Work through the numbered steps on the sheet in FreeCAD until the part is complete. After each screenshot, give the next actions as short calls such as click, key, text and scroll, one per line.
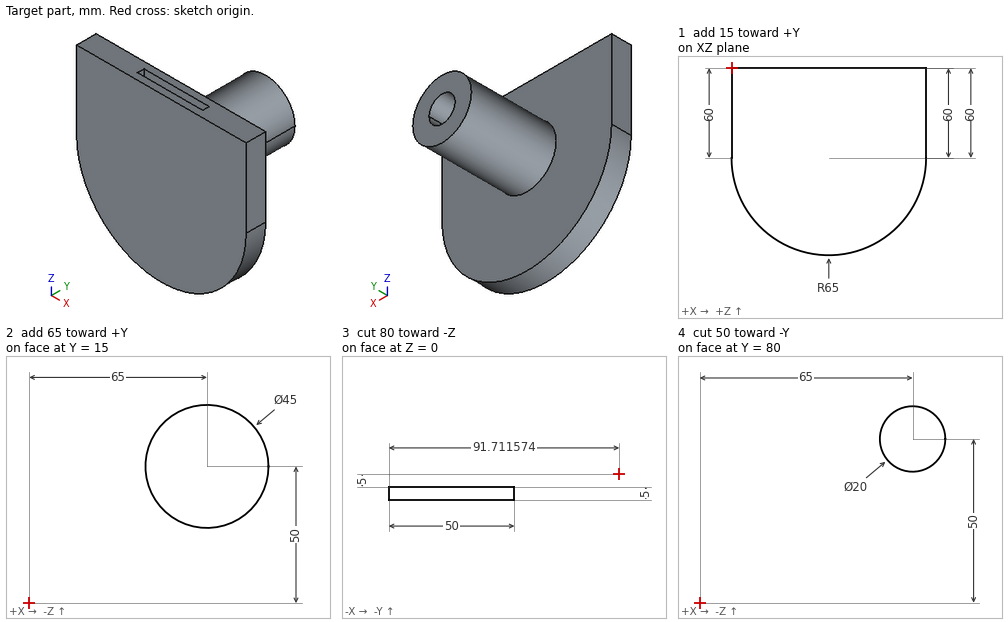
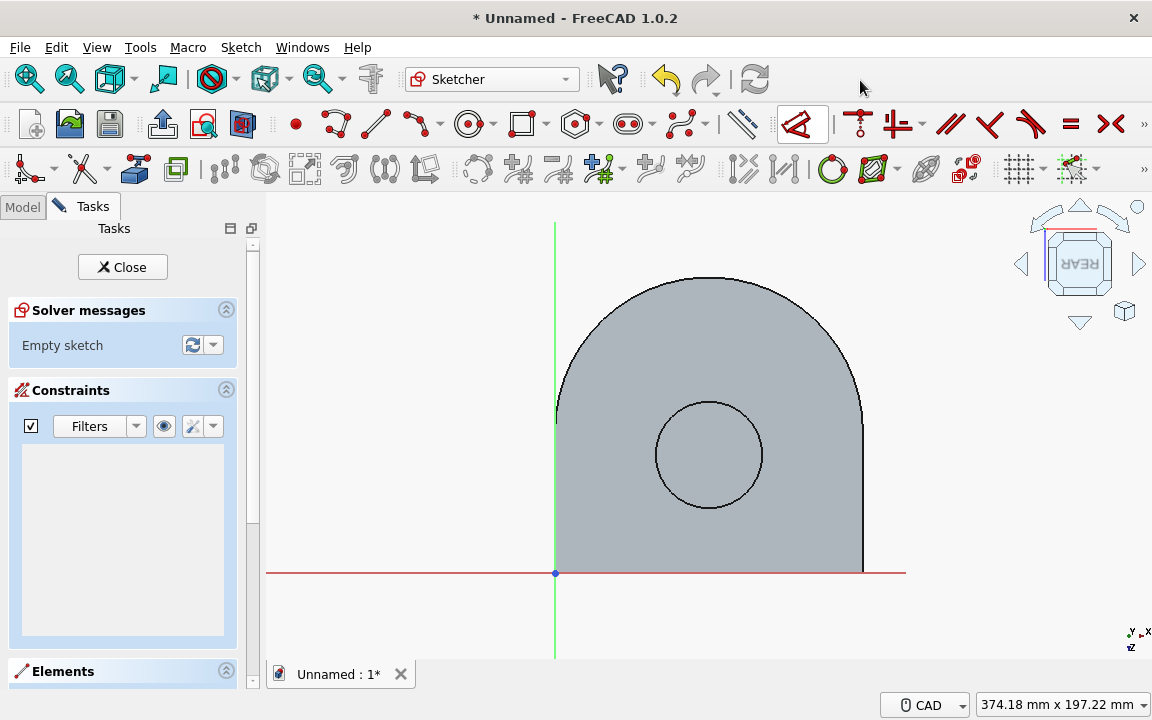
scroll(723, 461, up, 9)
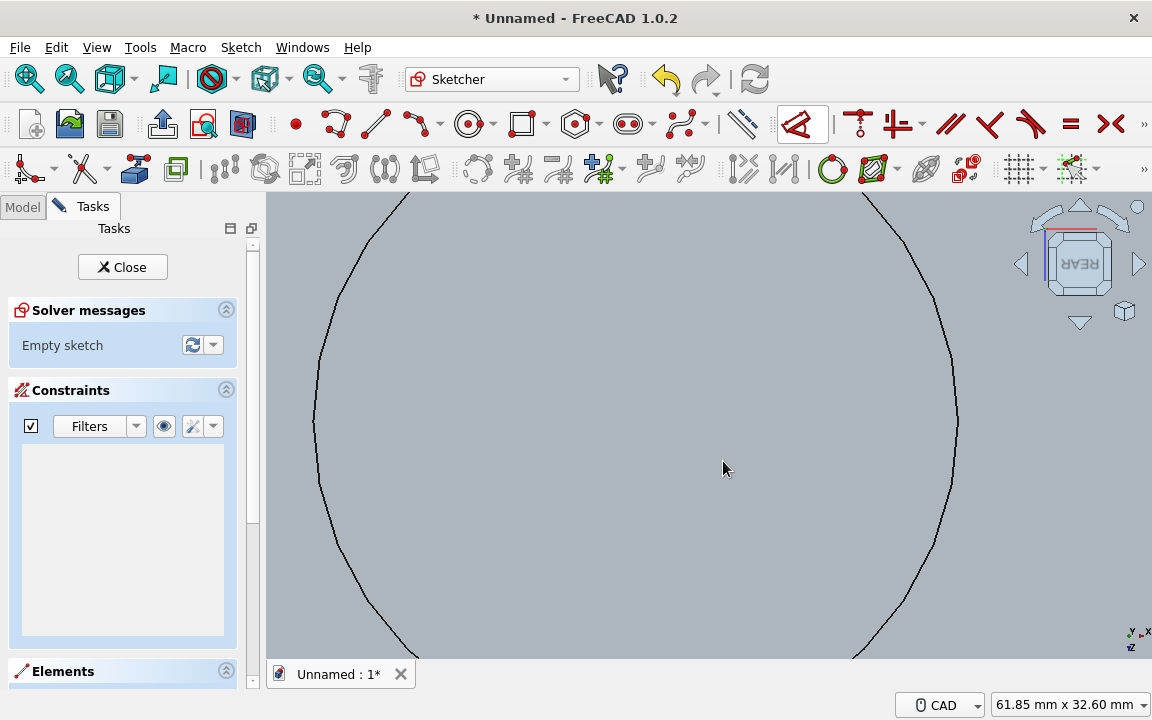
click(470, 124)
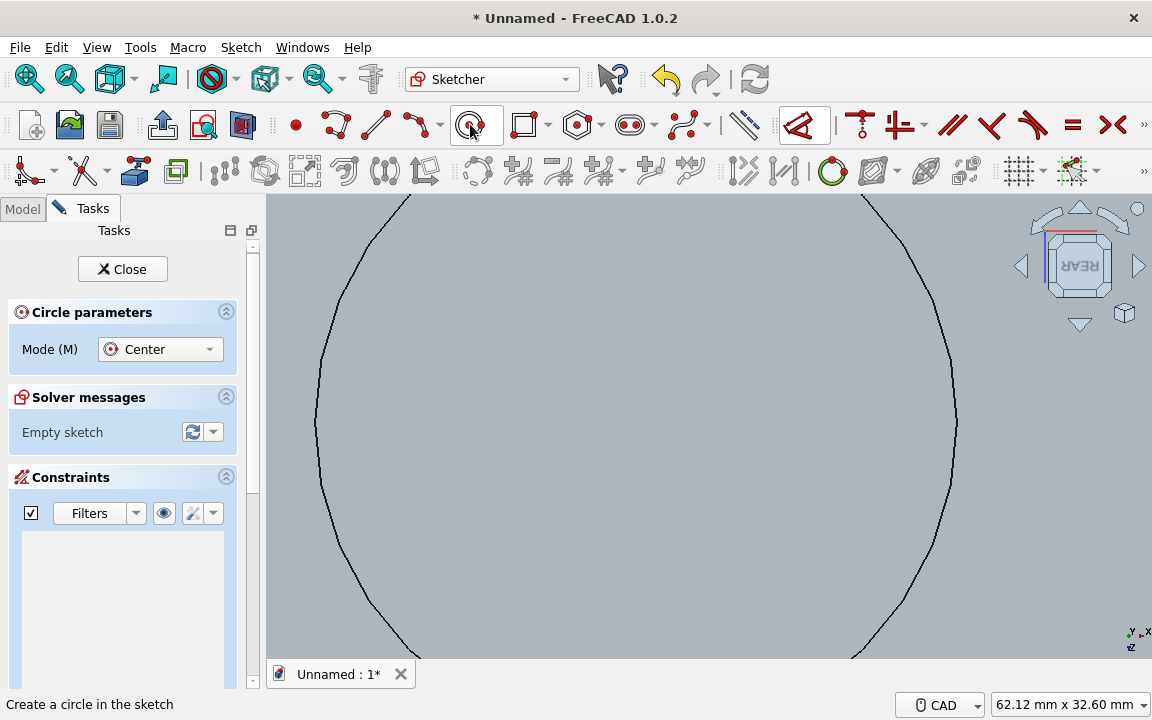
click(636, 423)
move(737, 322)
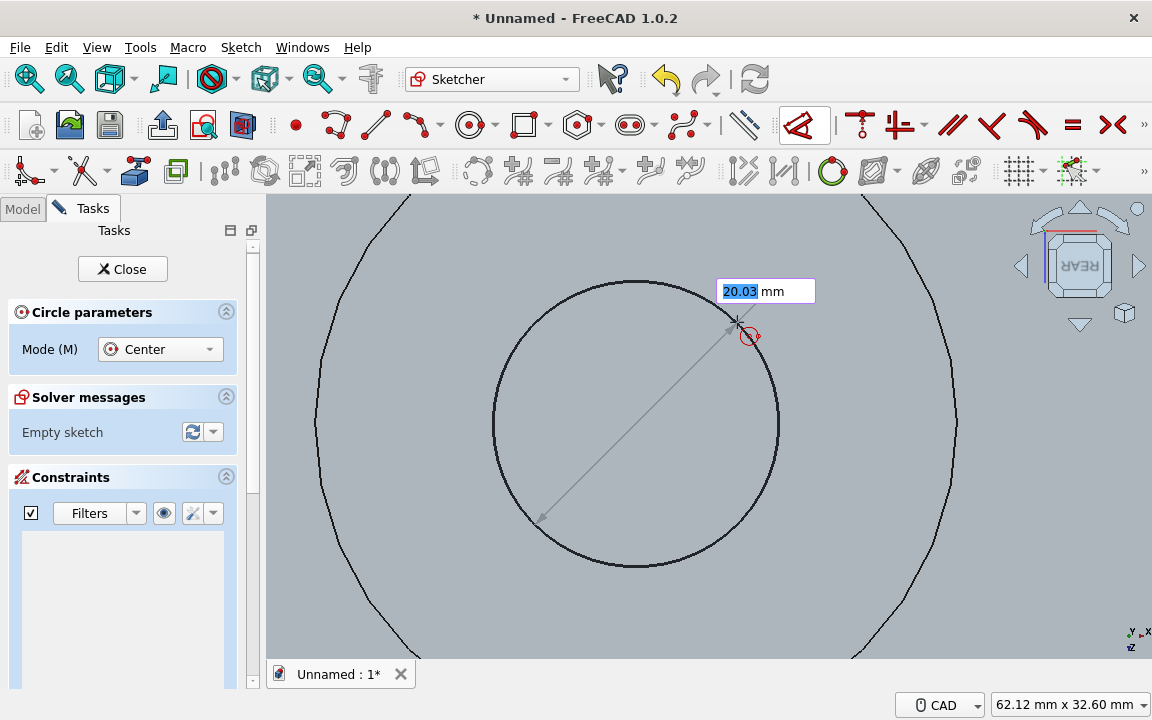
text(20)
key(Return)
key(Escape)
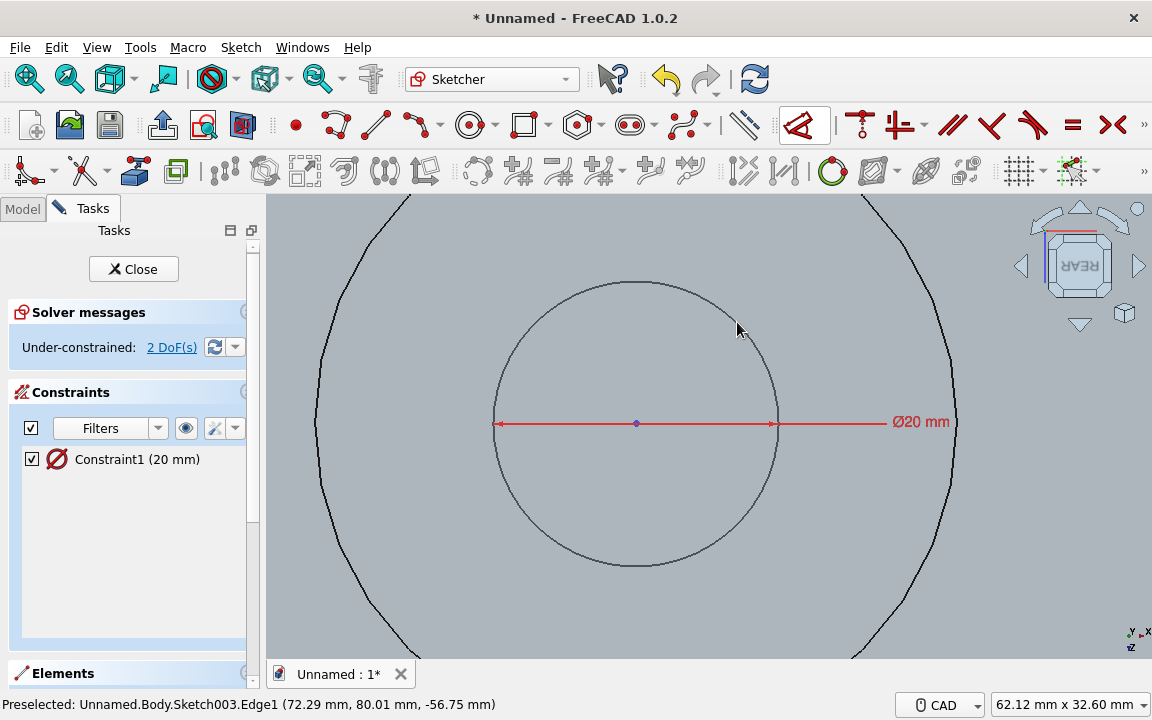
click(636, 424)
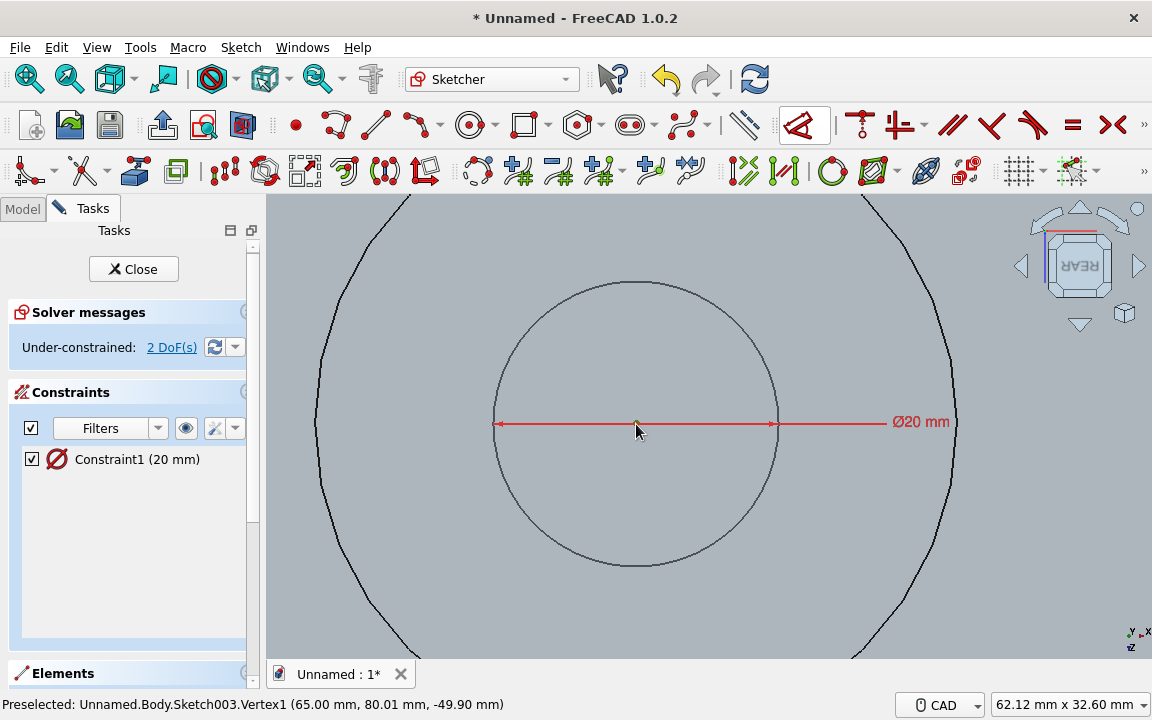
click(824, 126)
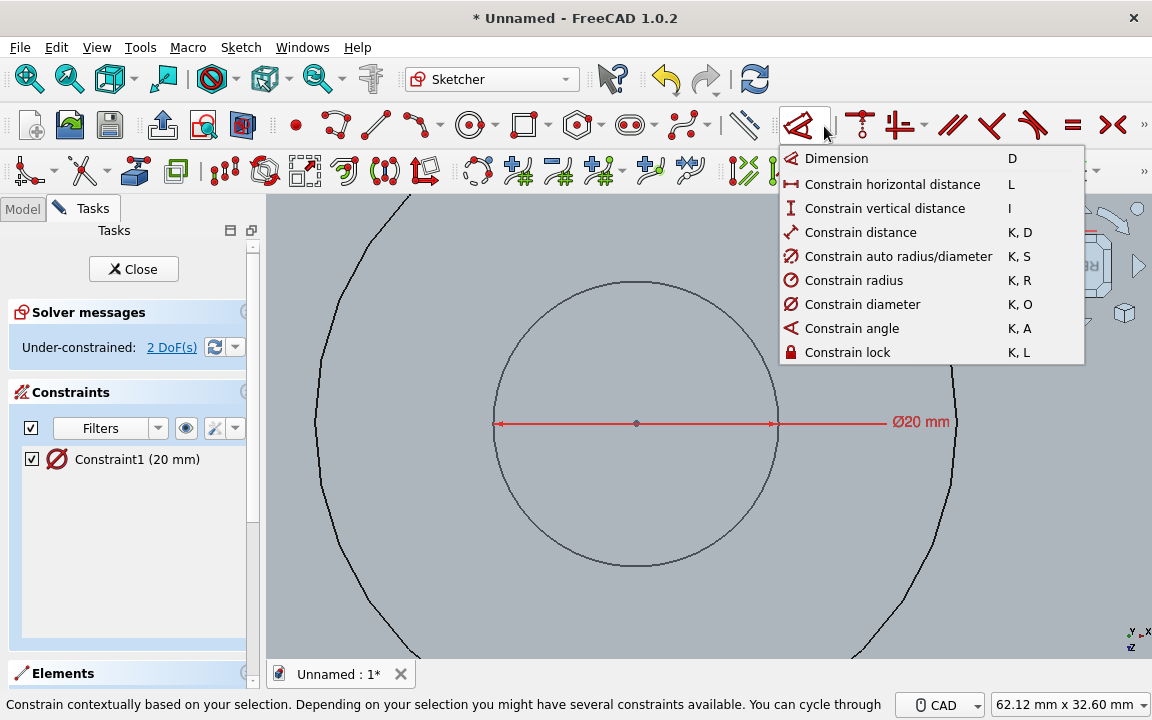
click(932, 184)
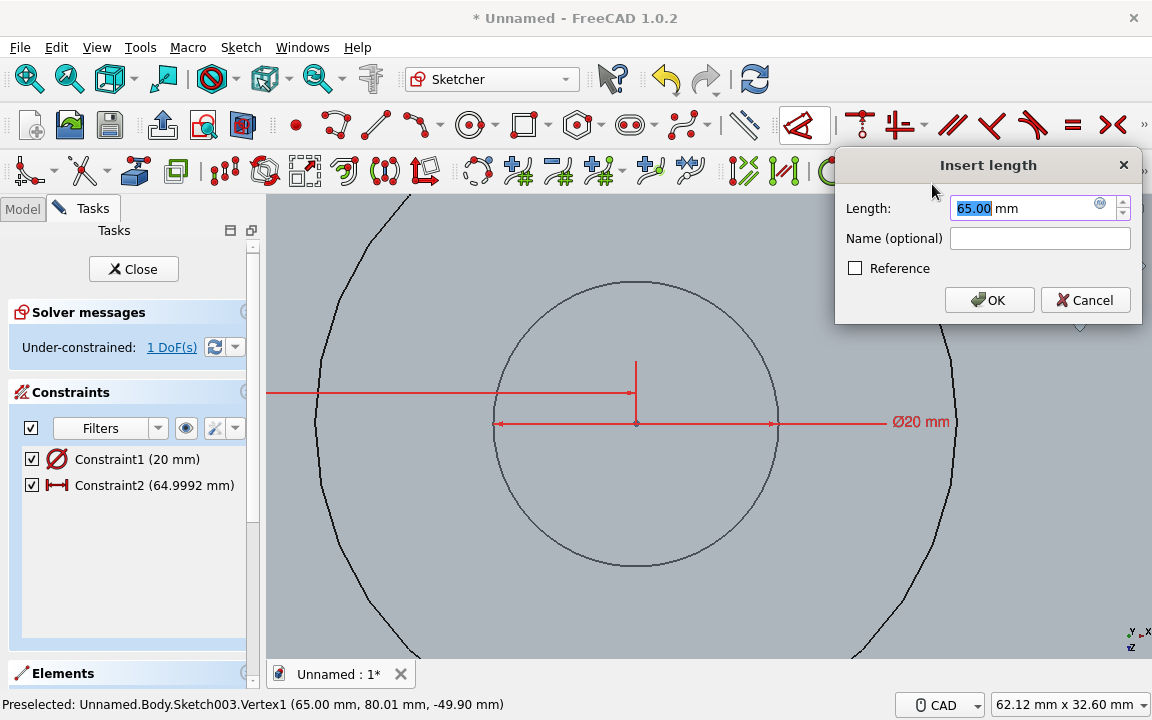
text(65)
key(Return)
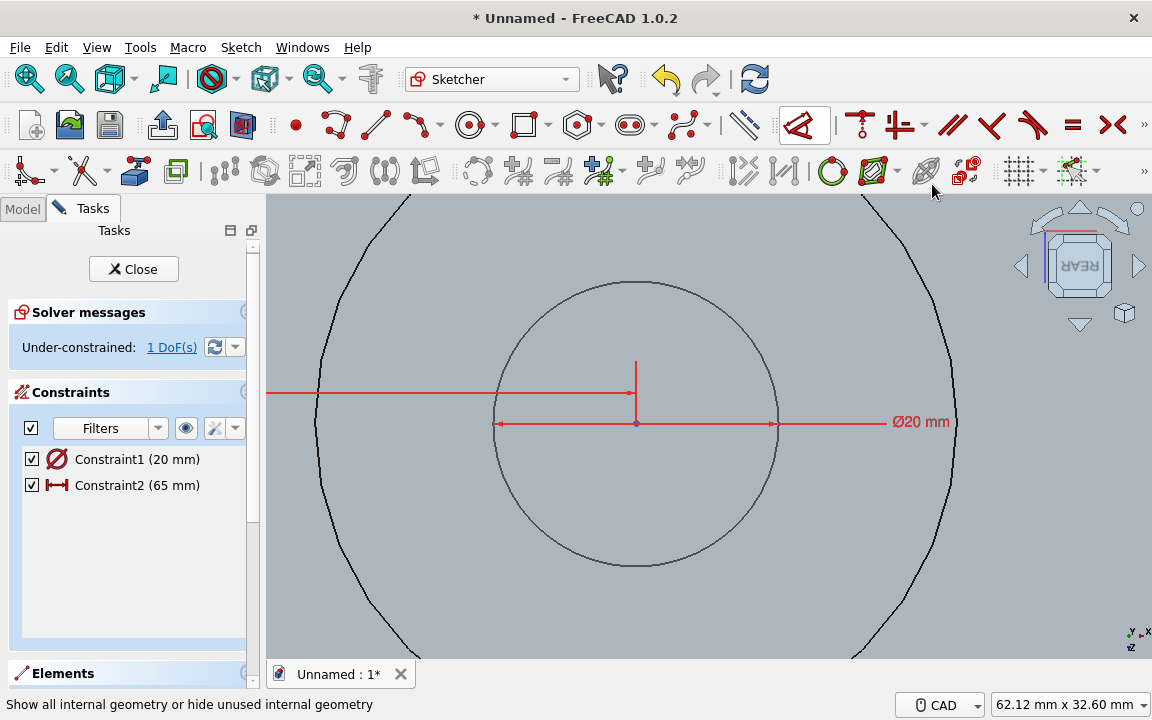
click(636, 424)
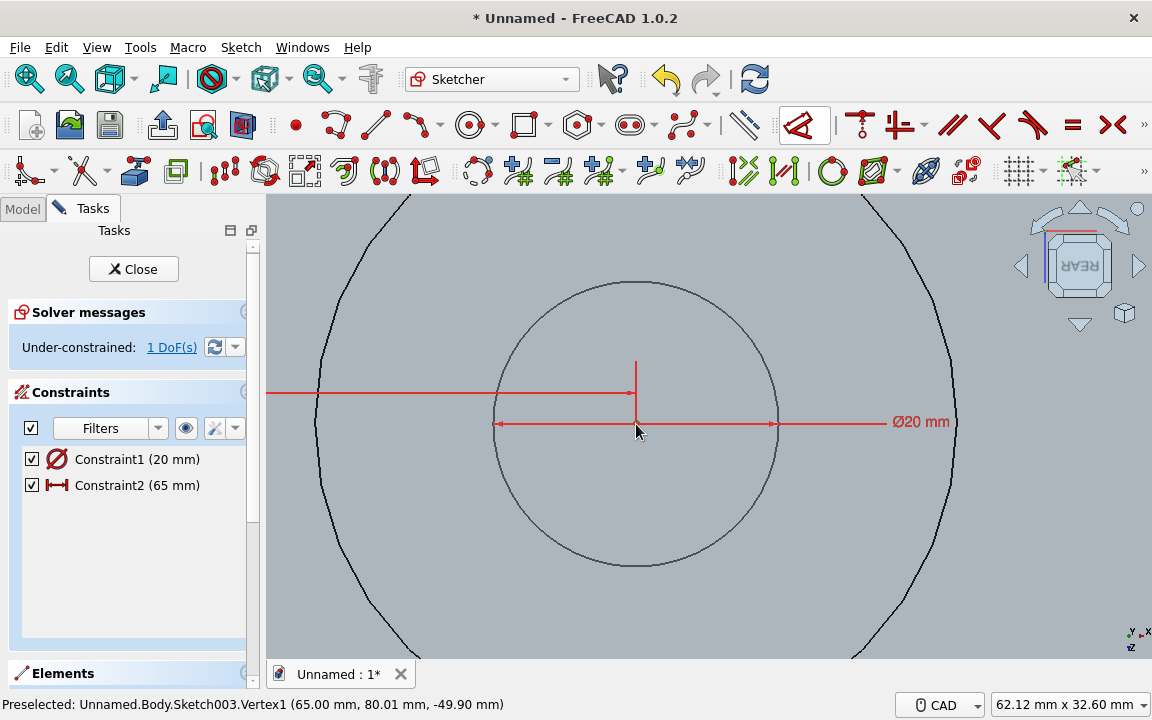
key(i)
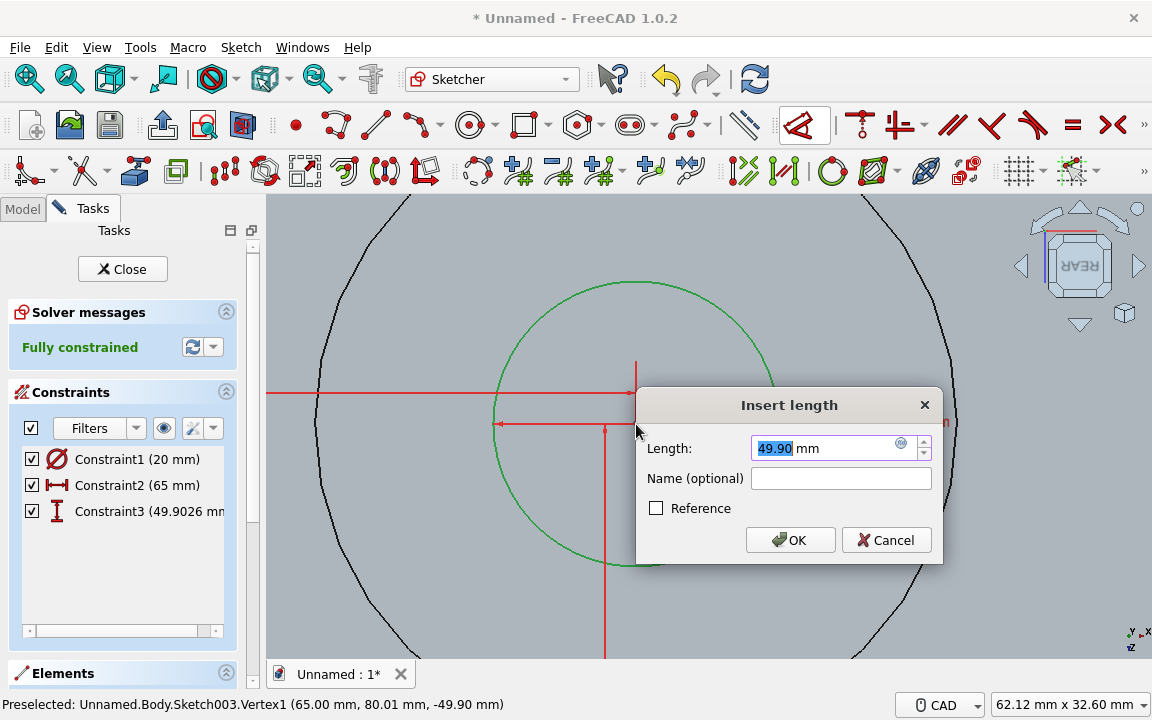
text(50)
key(Return)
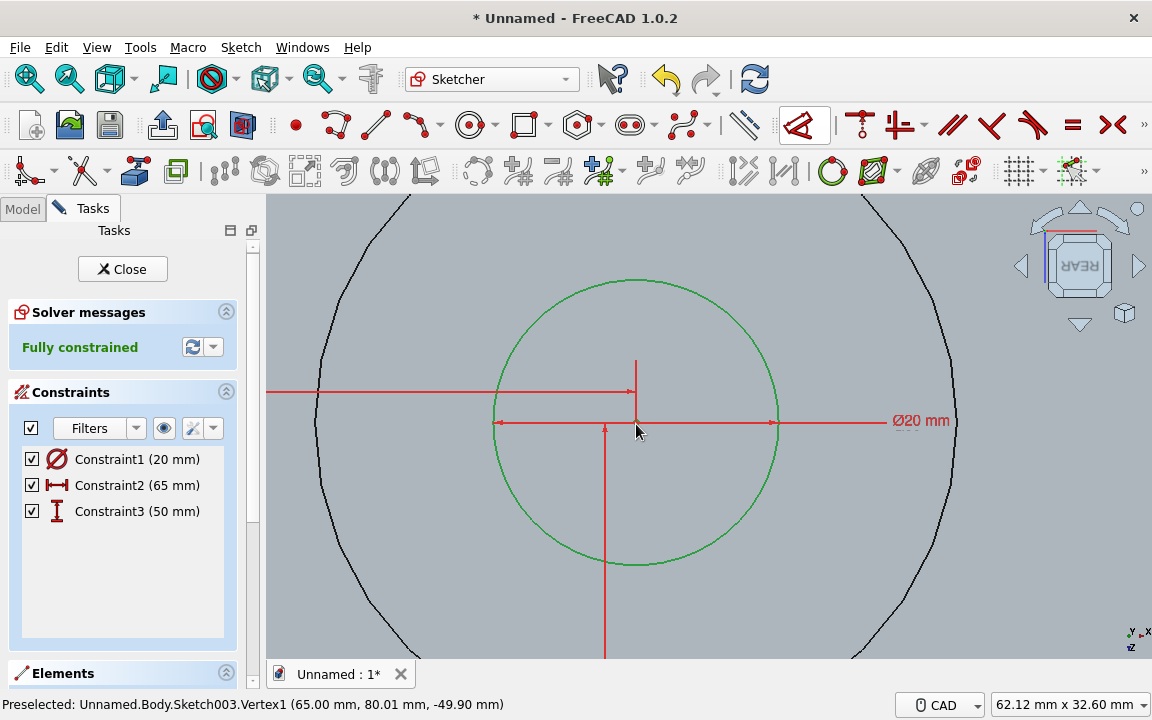
click(123, 269)